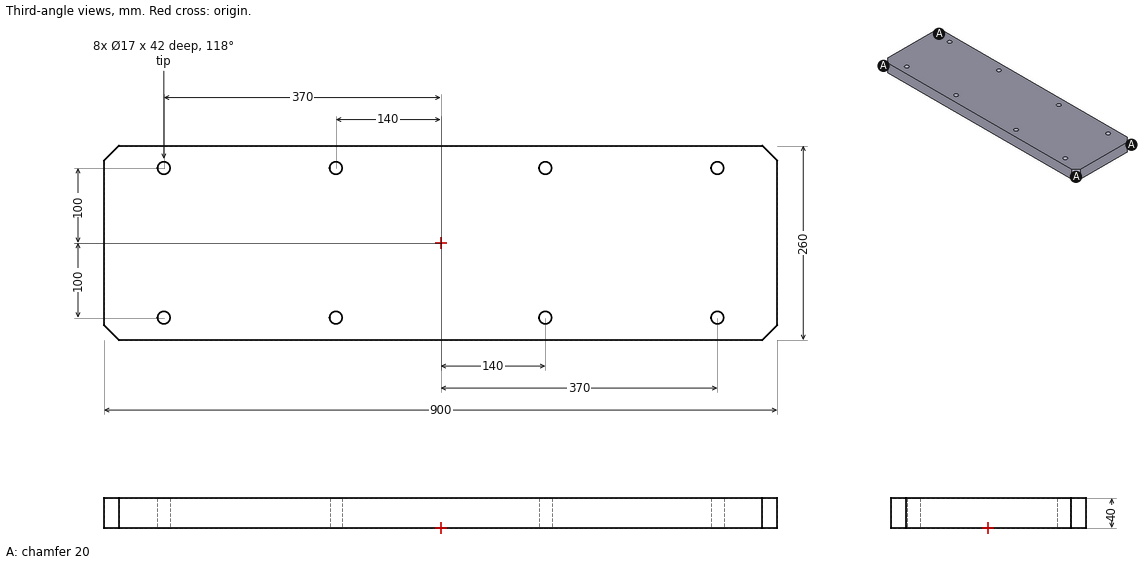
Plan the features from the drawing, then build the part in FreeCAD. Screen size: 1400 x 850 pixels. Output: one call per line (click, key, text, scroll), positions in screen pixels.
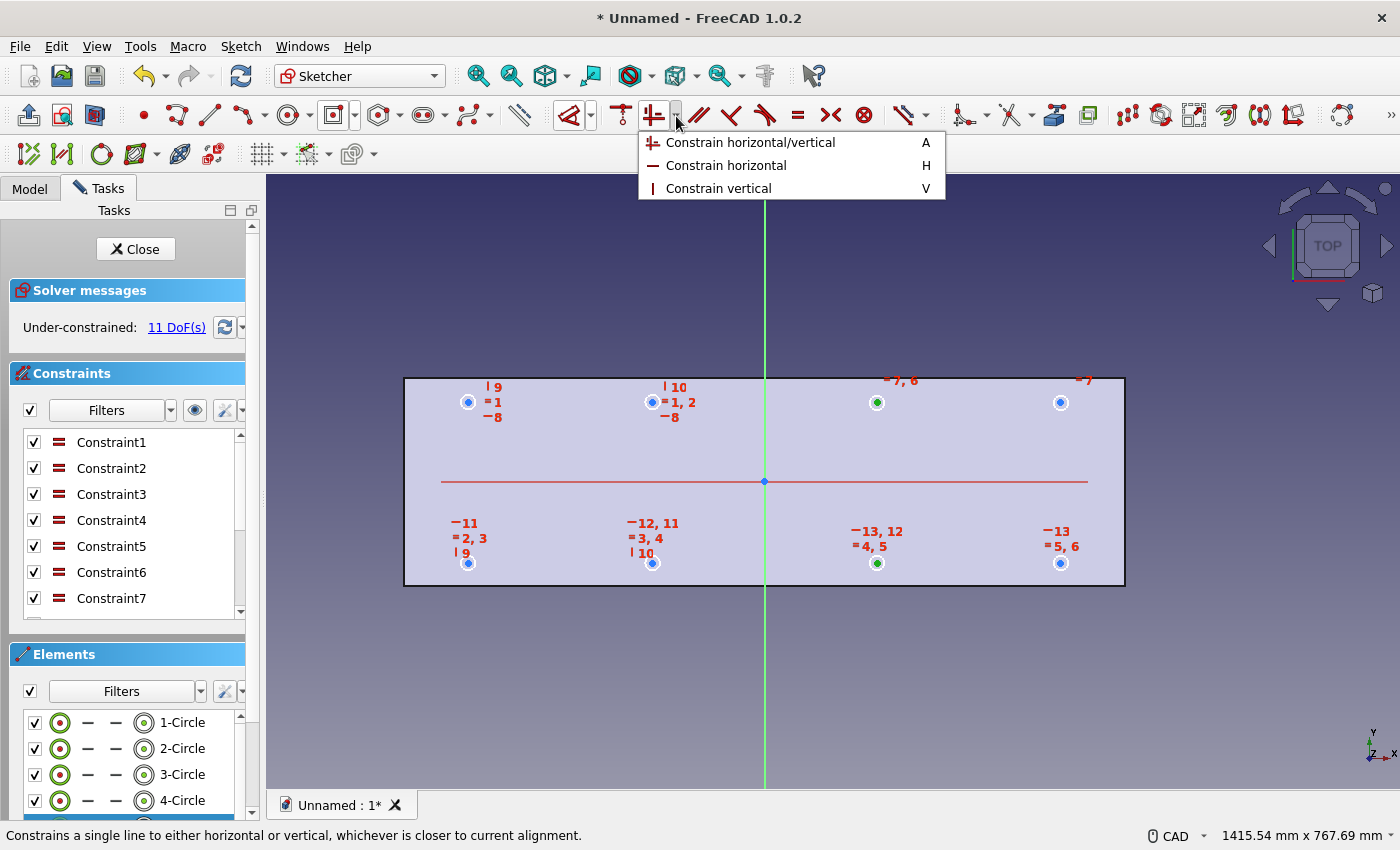
click(792, 188)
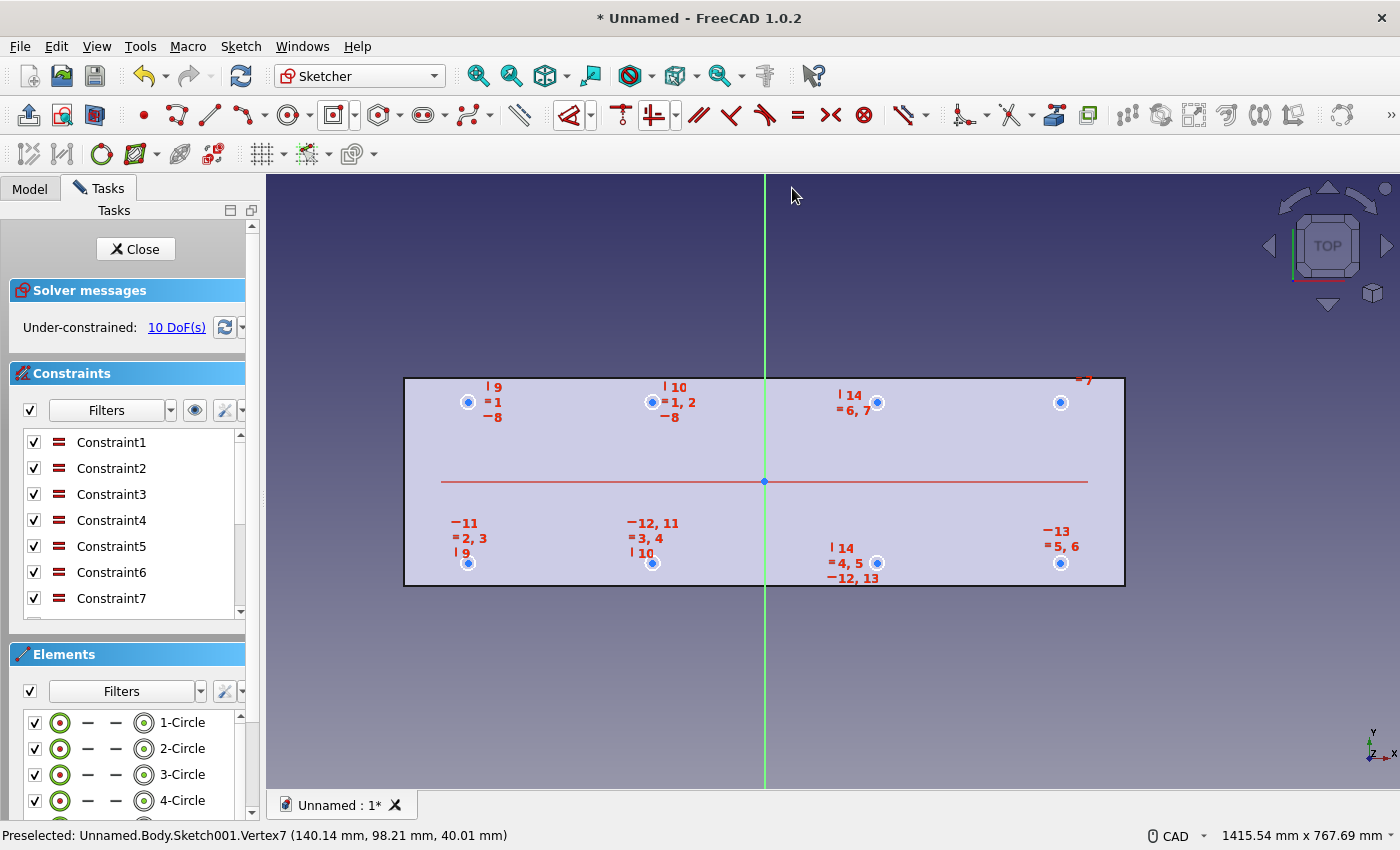
click(653, 402)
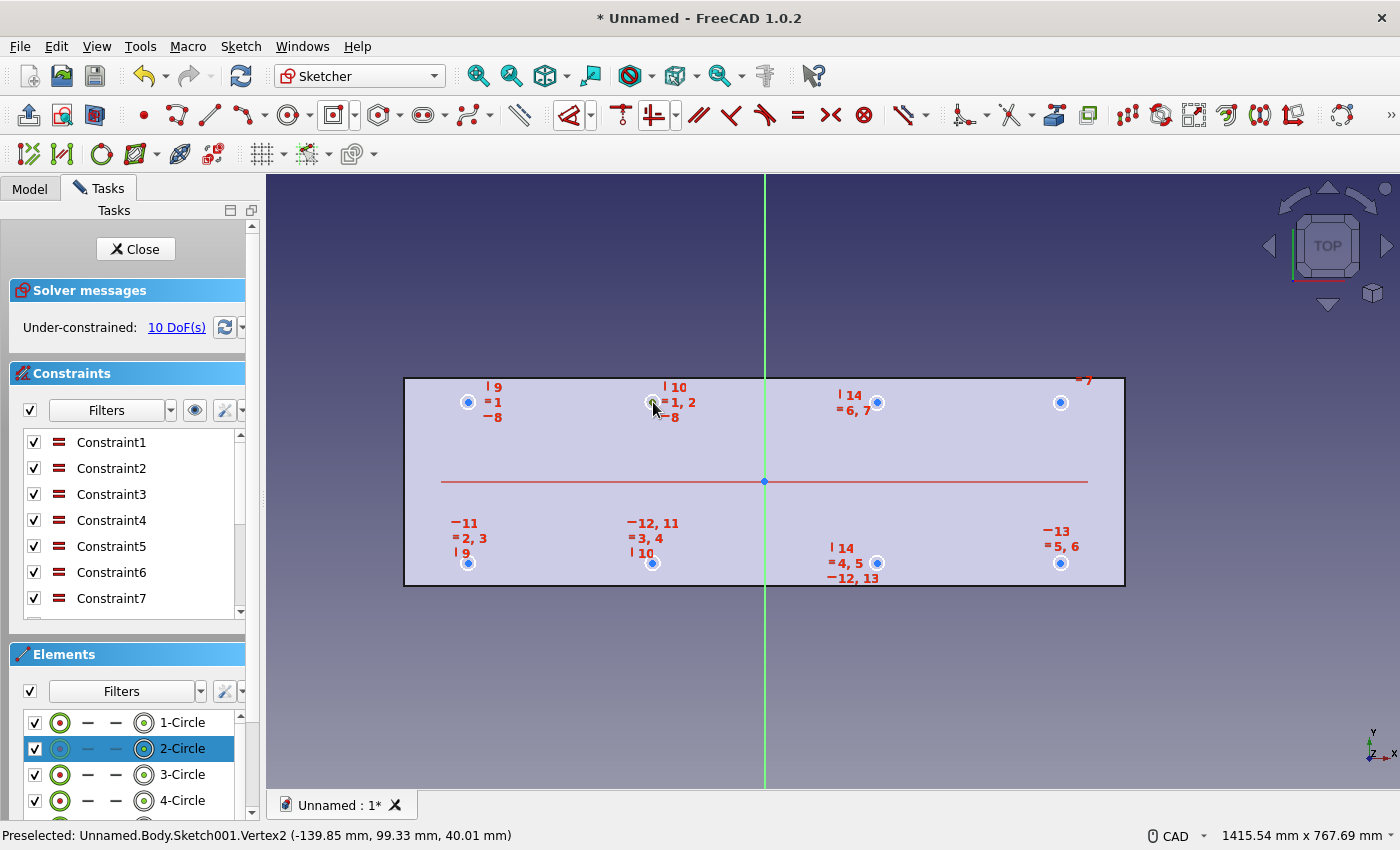
click(877, 403)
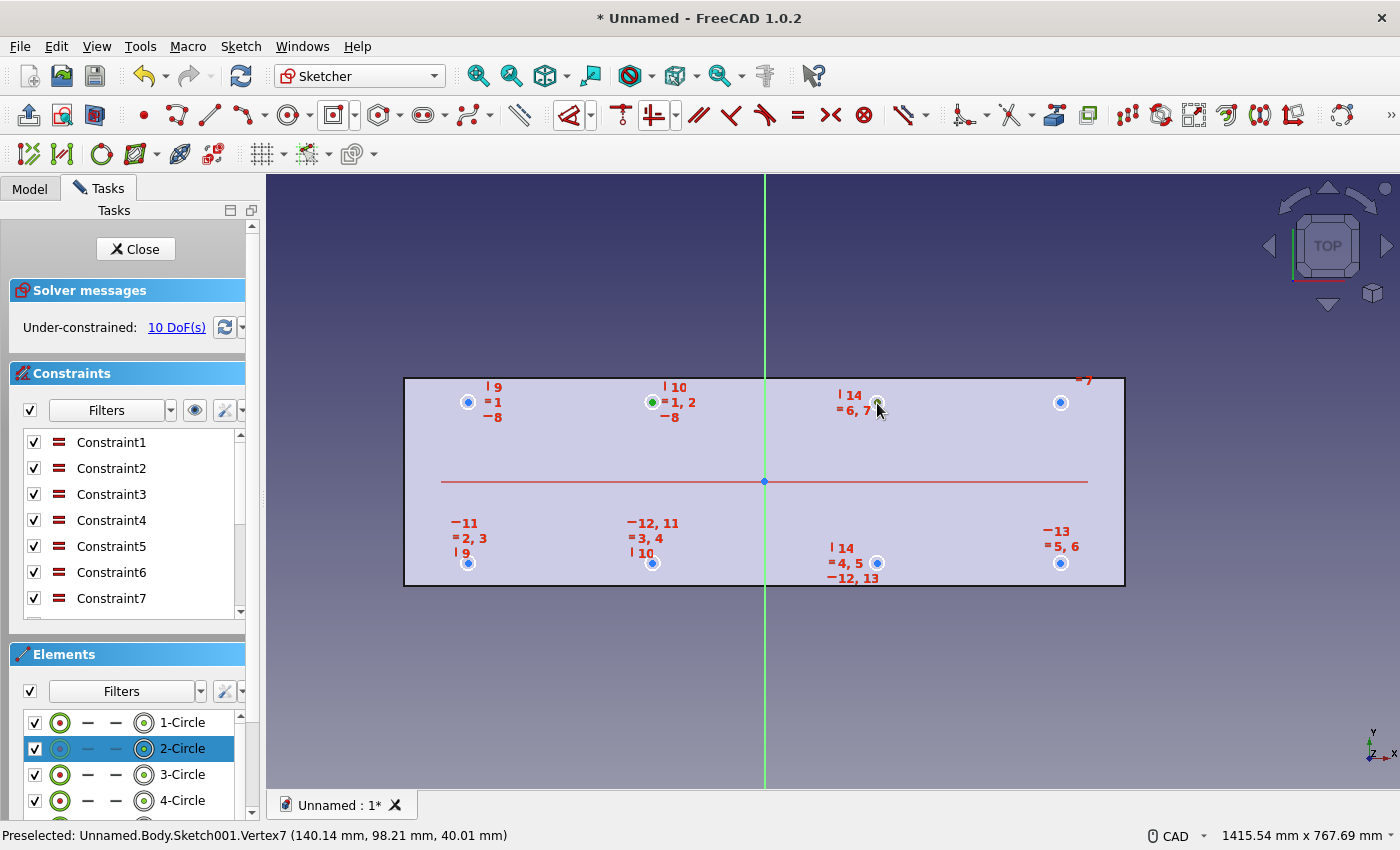
click(676, 116)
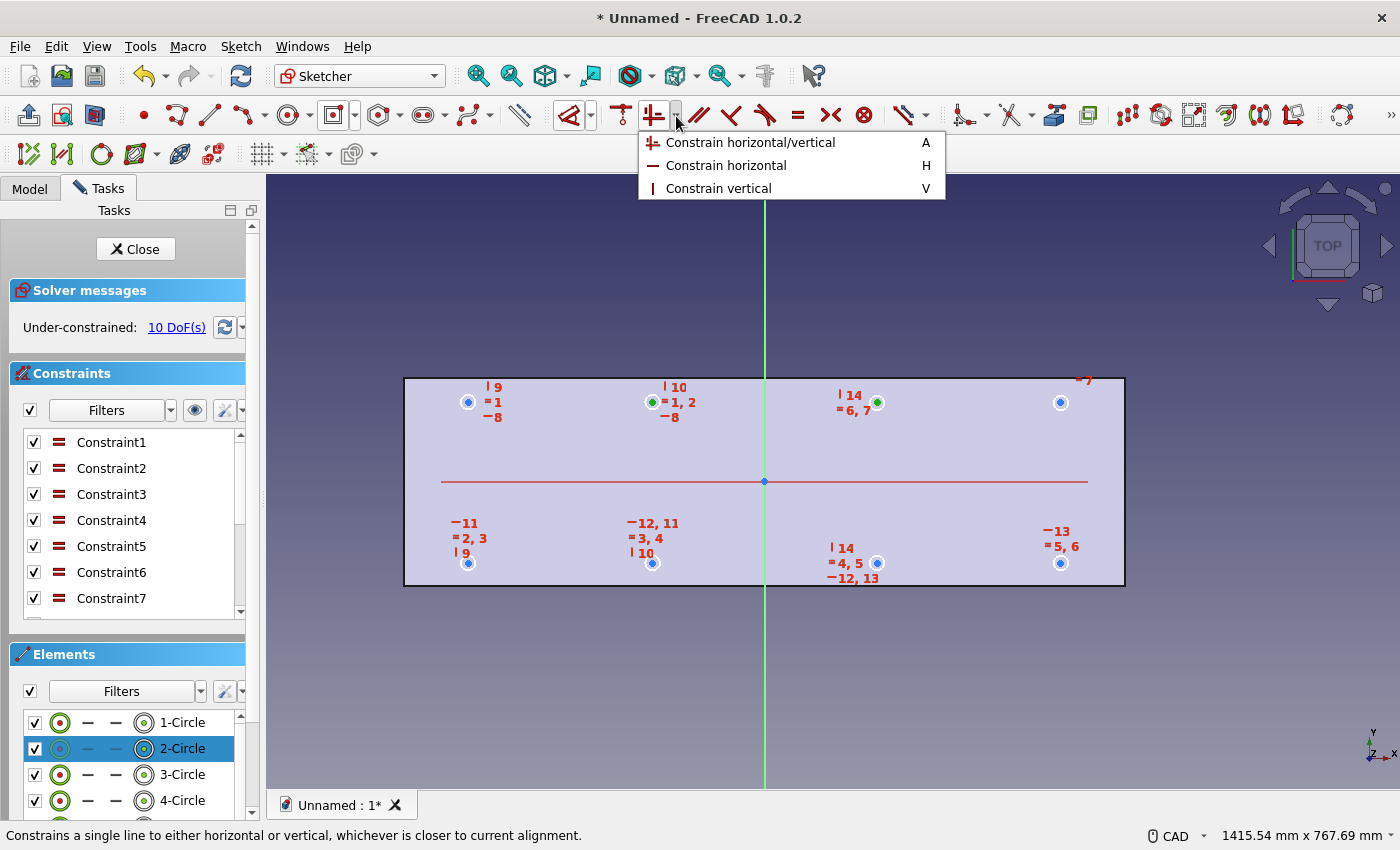
click(792, 166)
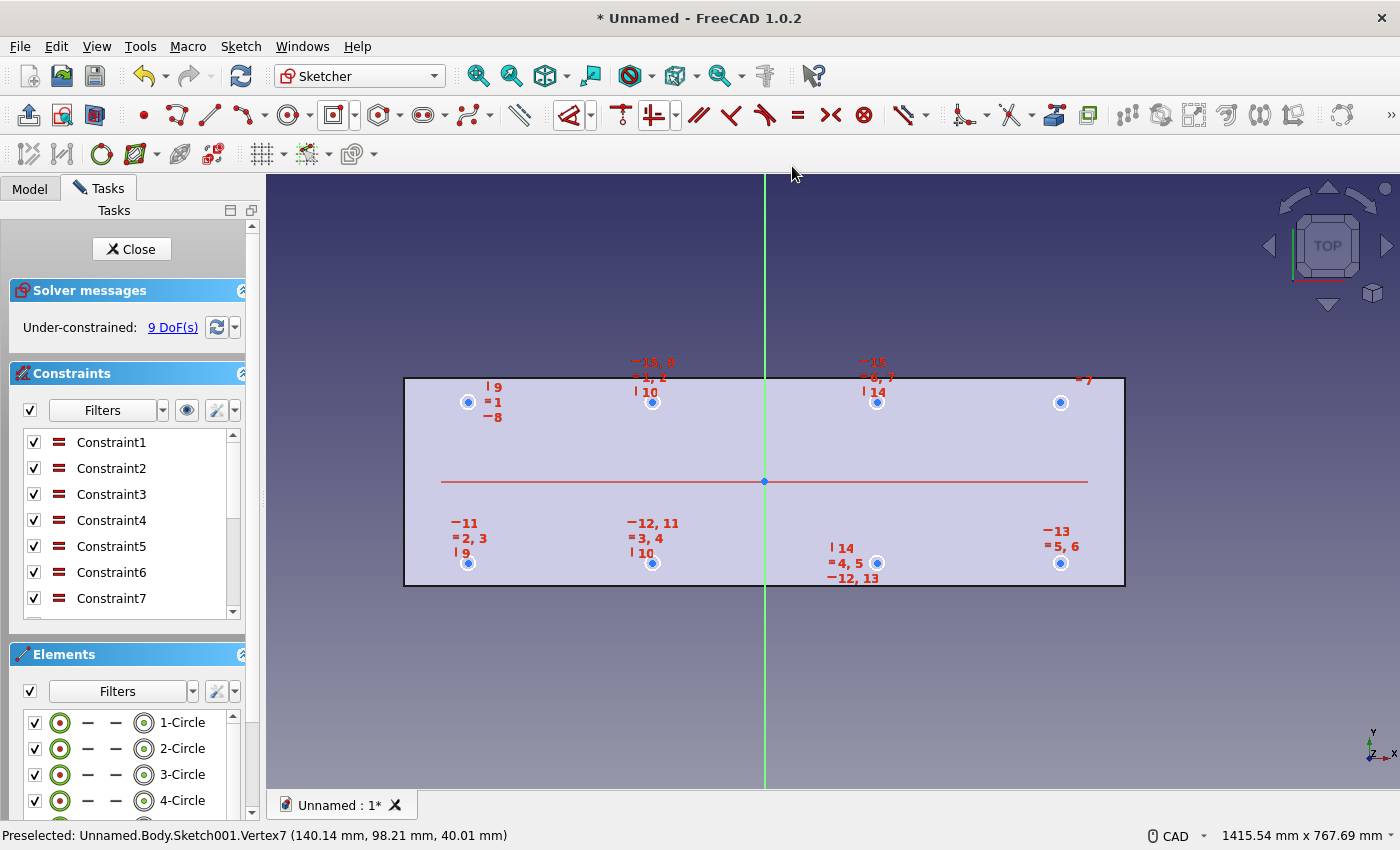
click(1061, 563)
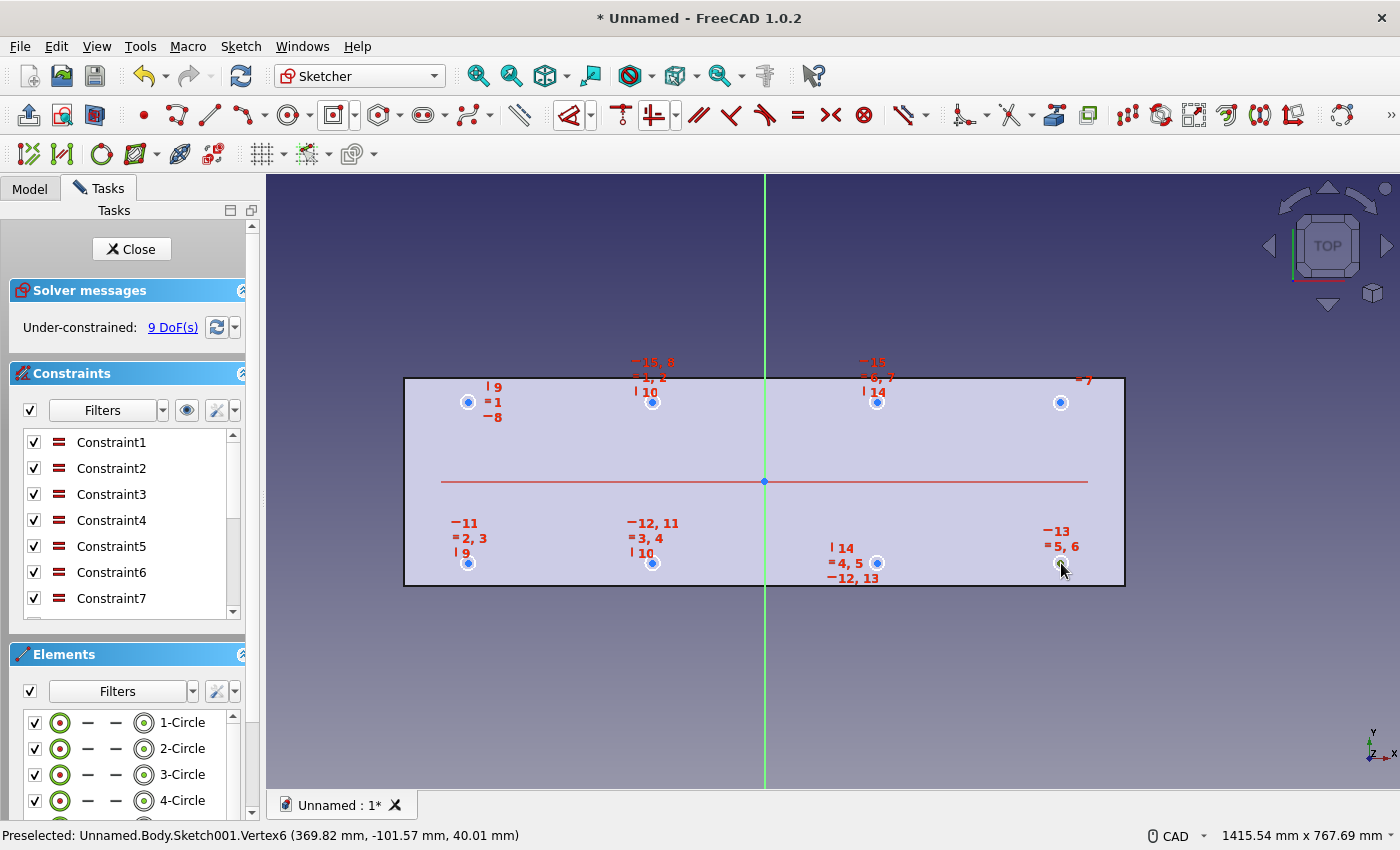
click(1061, 403)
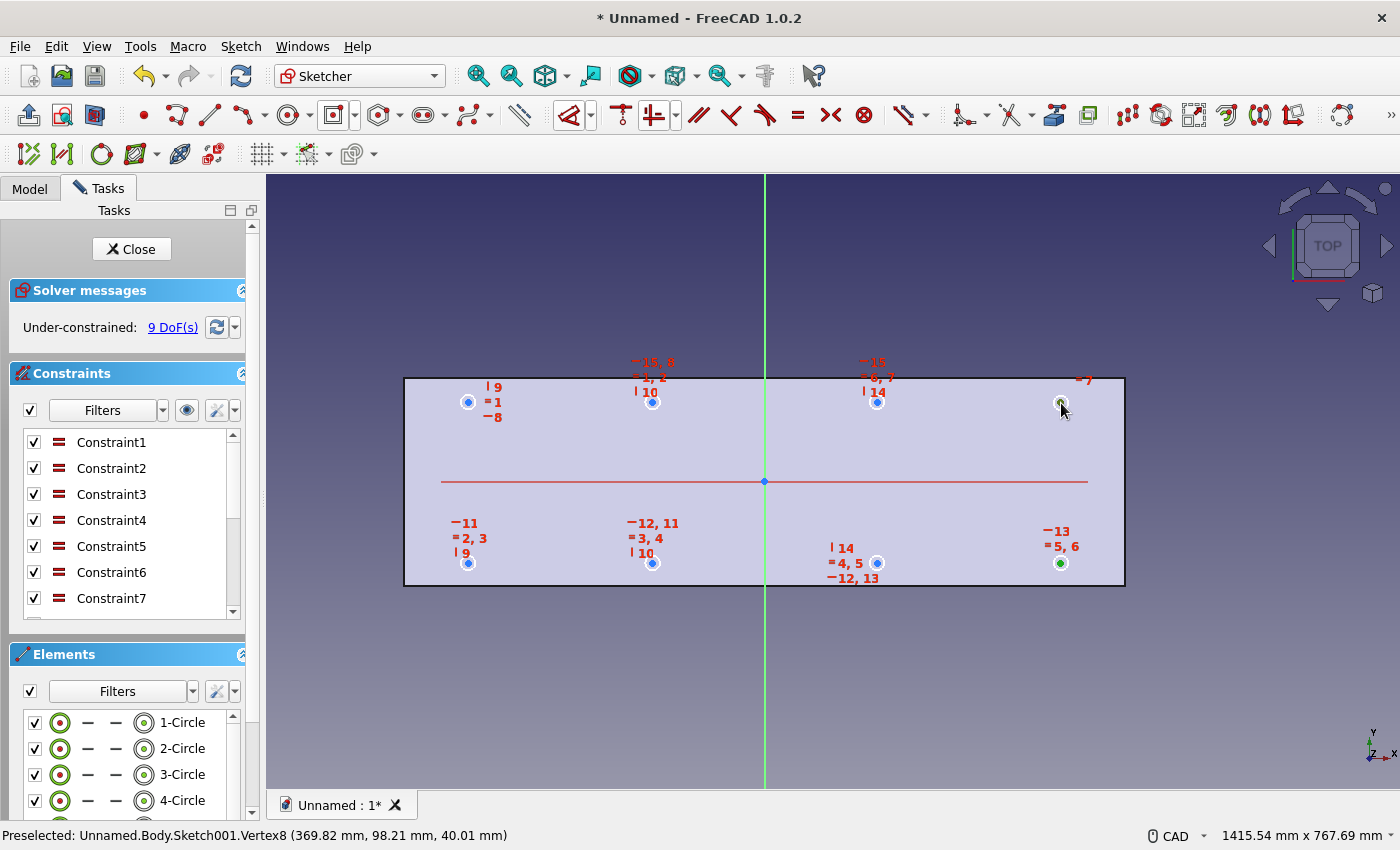
click(676, 116)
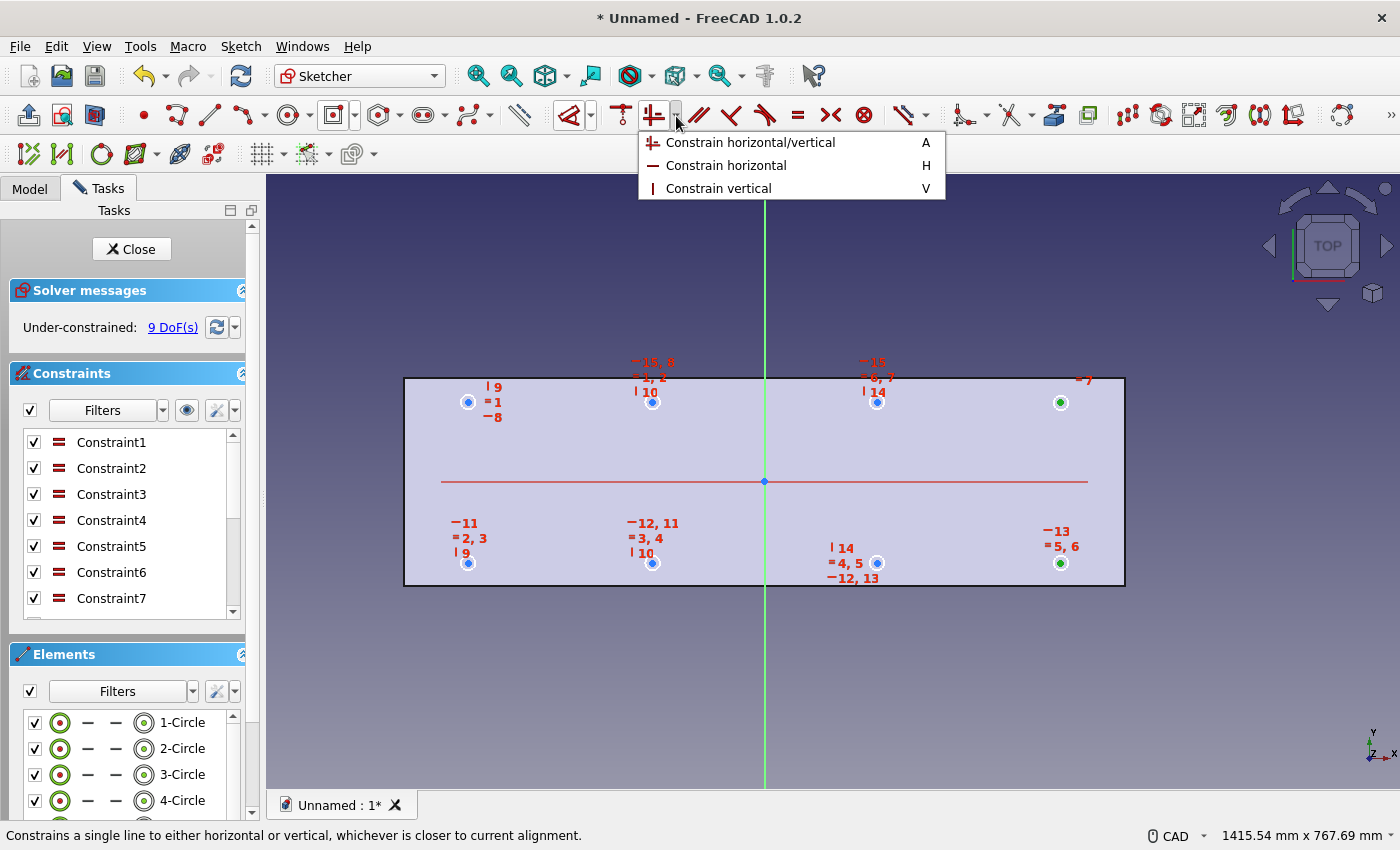
click(792, 188)